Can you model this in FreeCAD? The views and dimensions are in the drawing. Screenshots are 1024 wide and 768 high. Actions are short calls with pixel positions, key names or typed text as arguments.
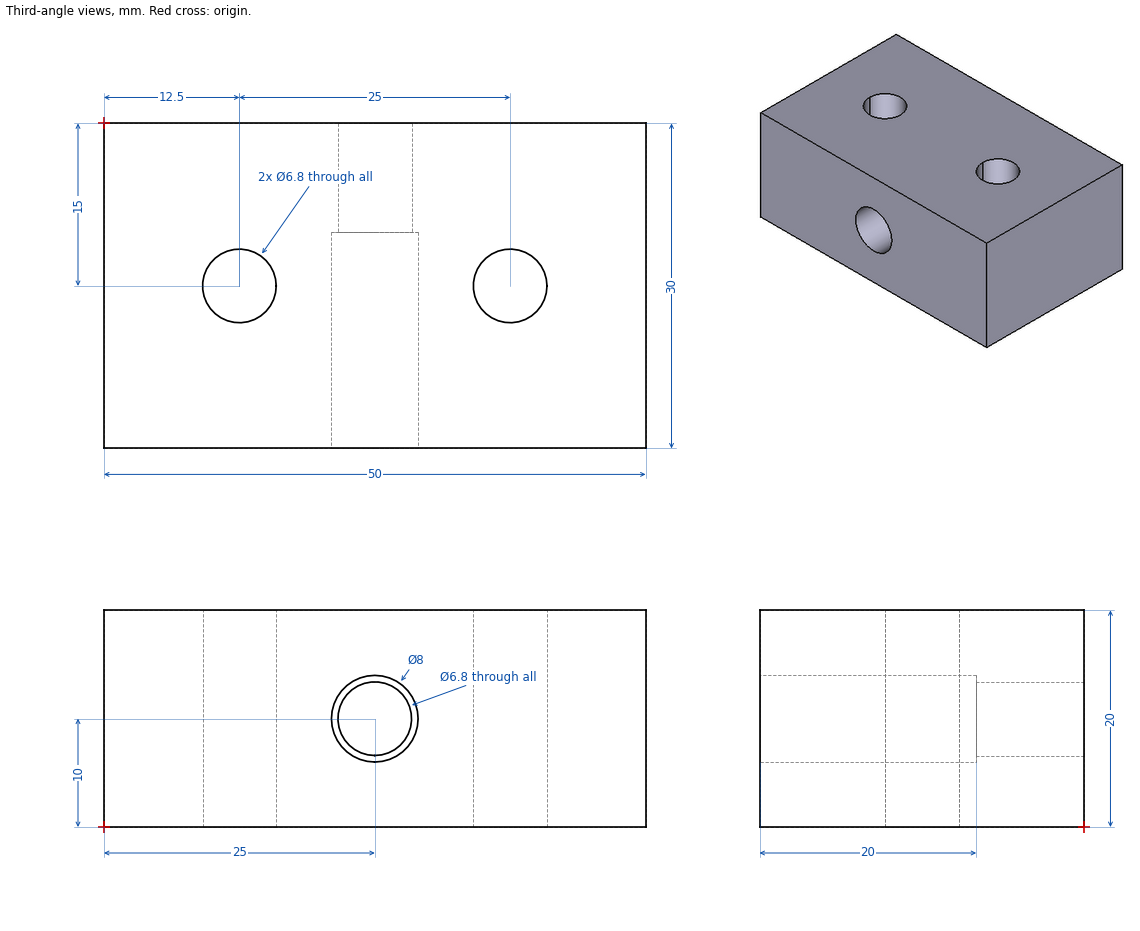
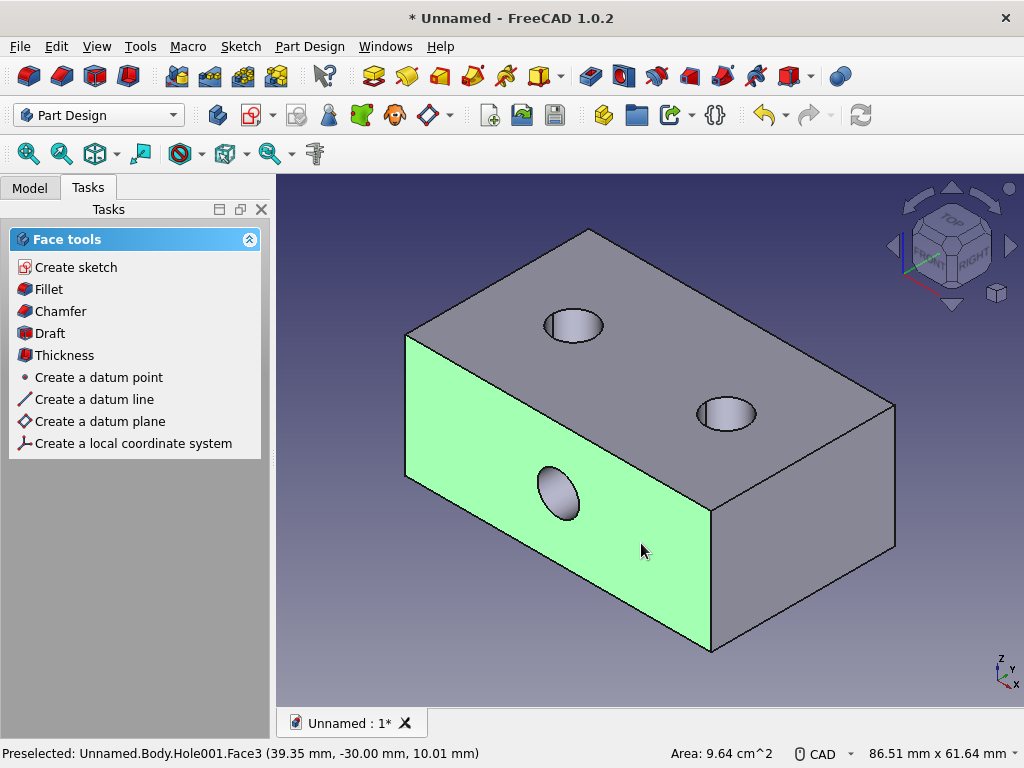
click(250, 116)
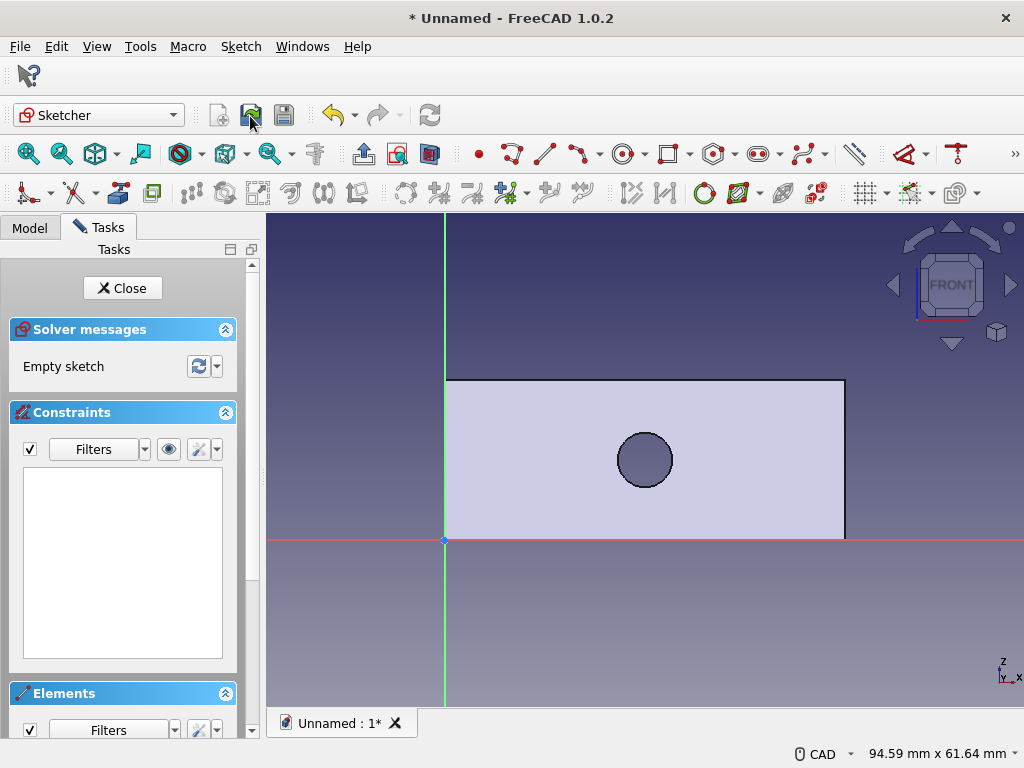
scroll(662, 460, up, 8)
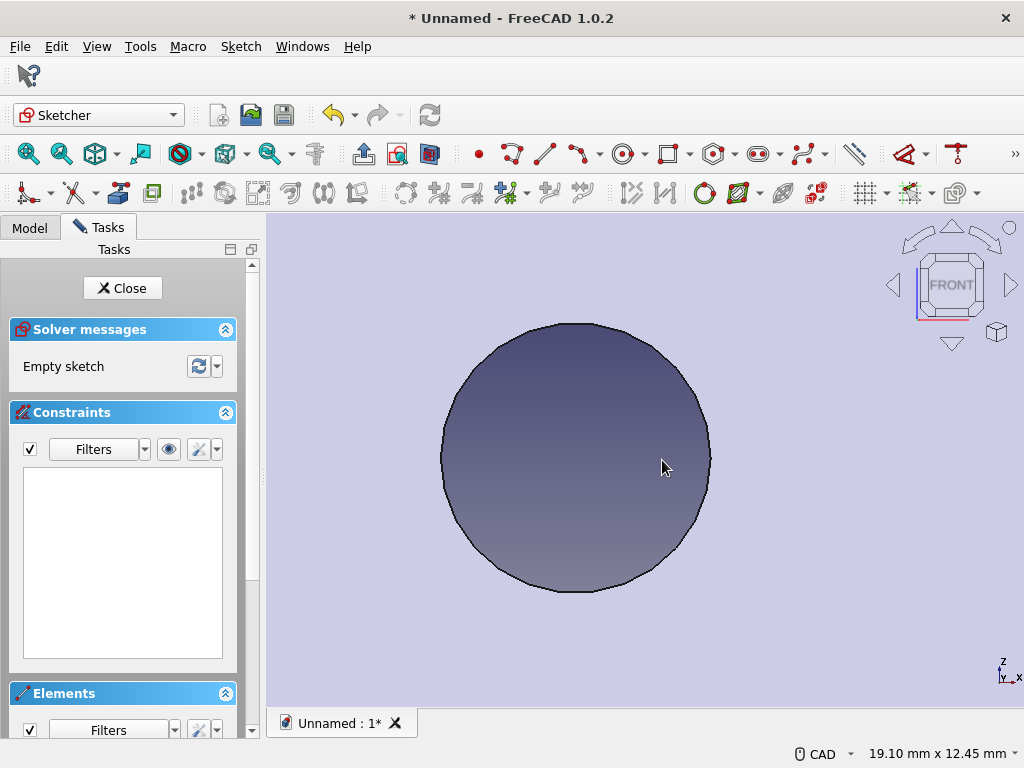
click(622, 154)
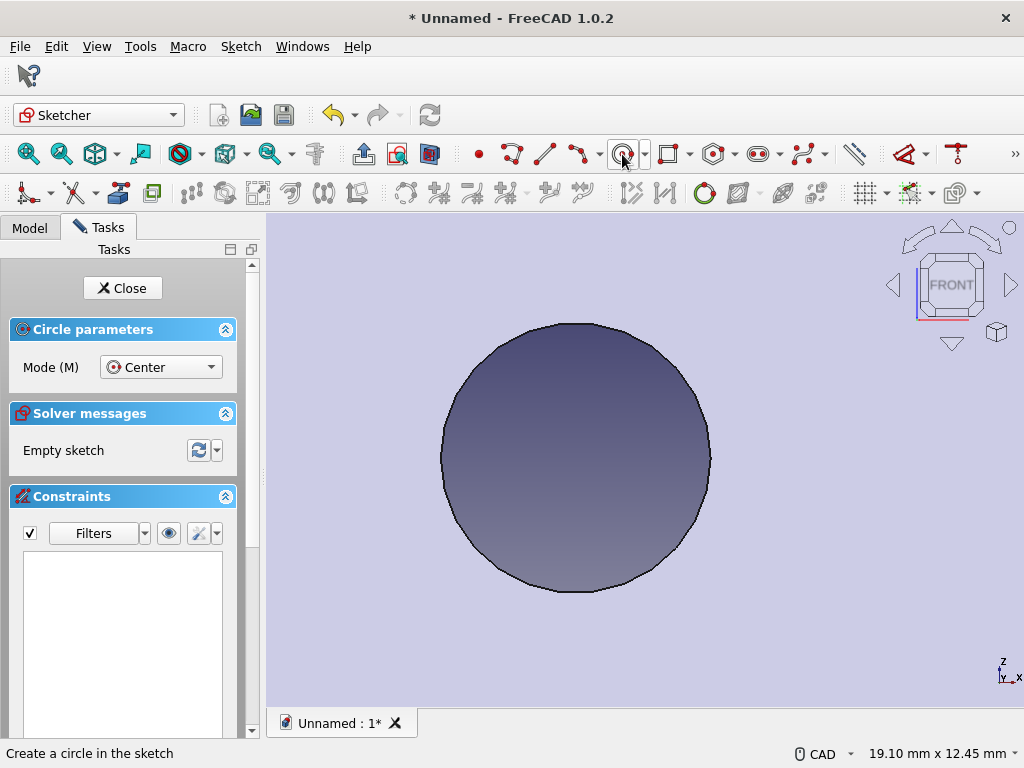
click(576, 458)
move(688, 346)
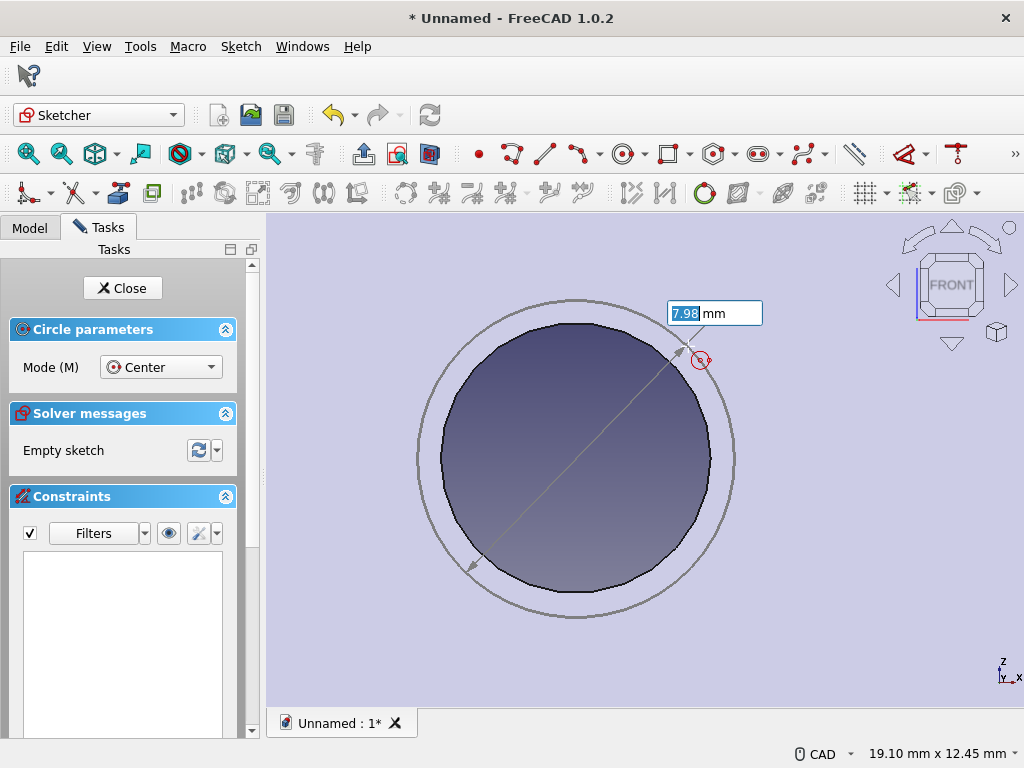
text(8)
key(Return)
key(Escape)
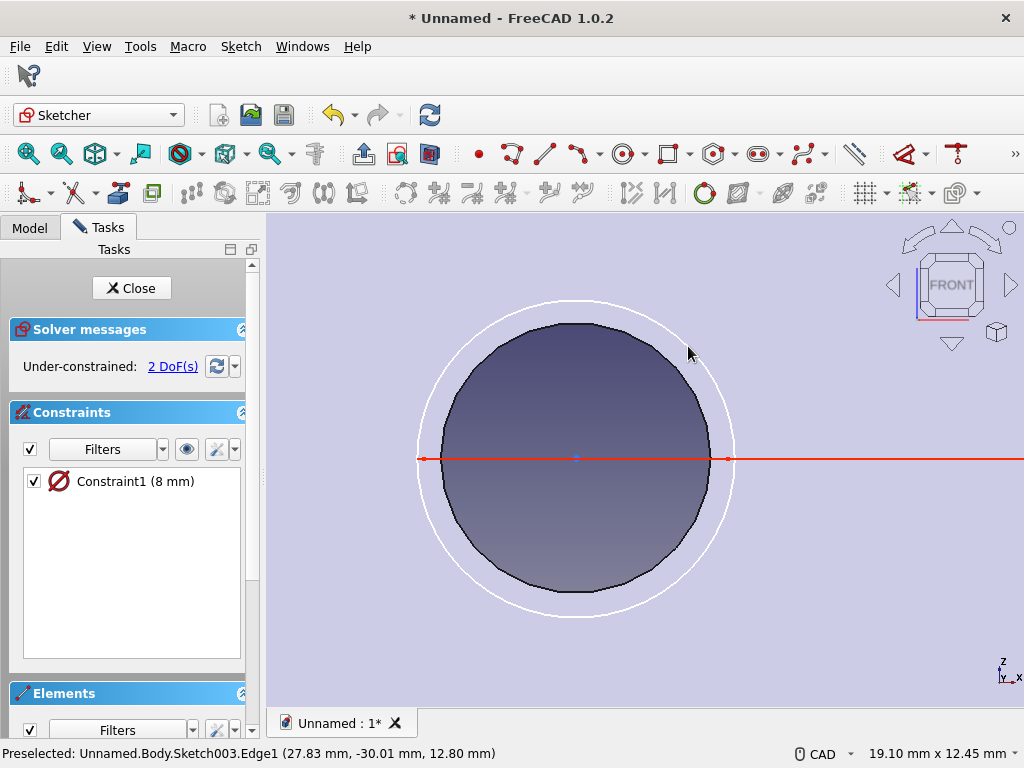
click(904, 154)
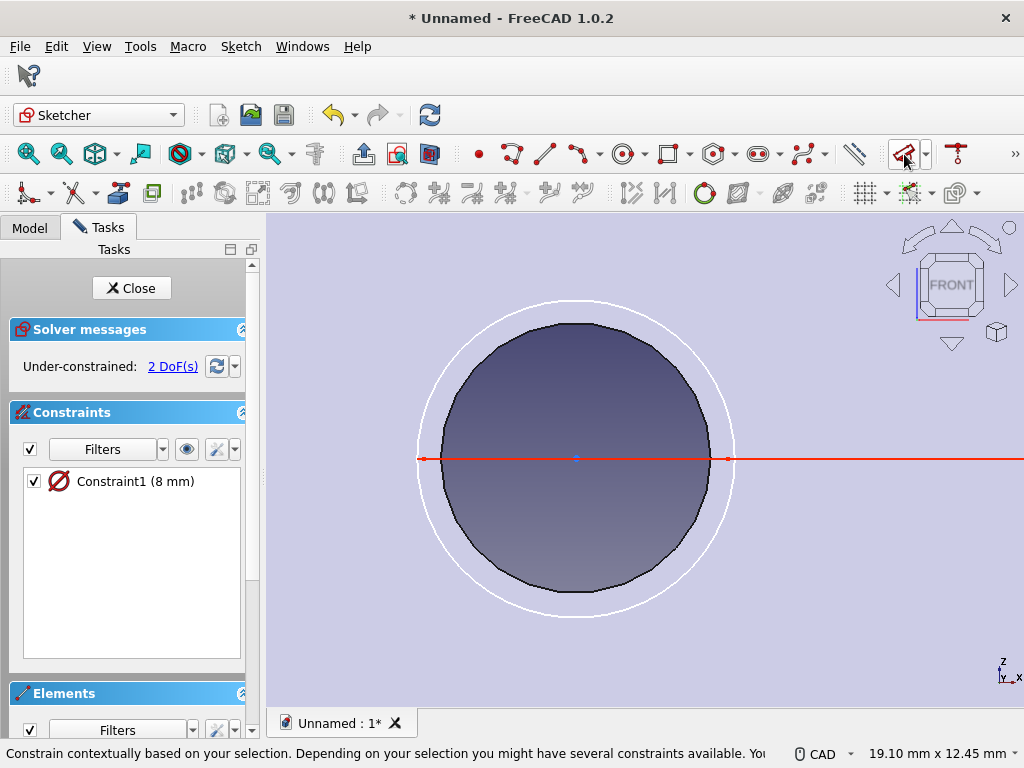
click(576, 459)
click(435, 425)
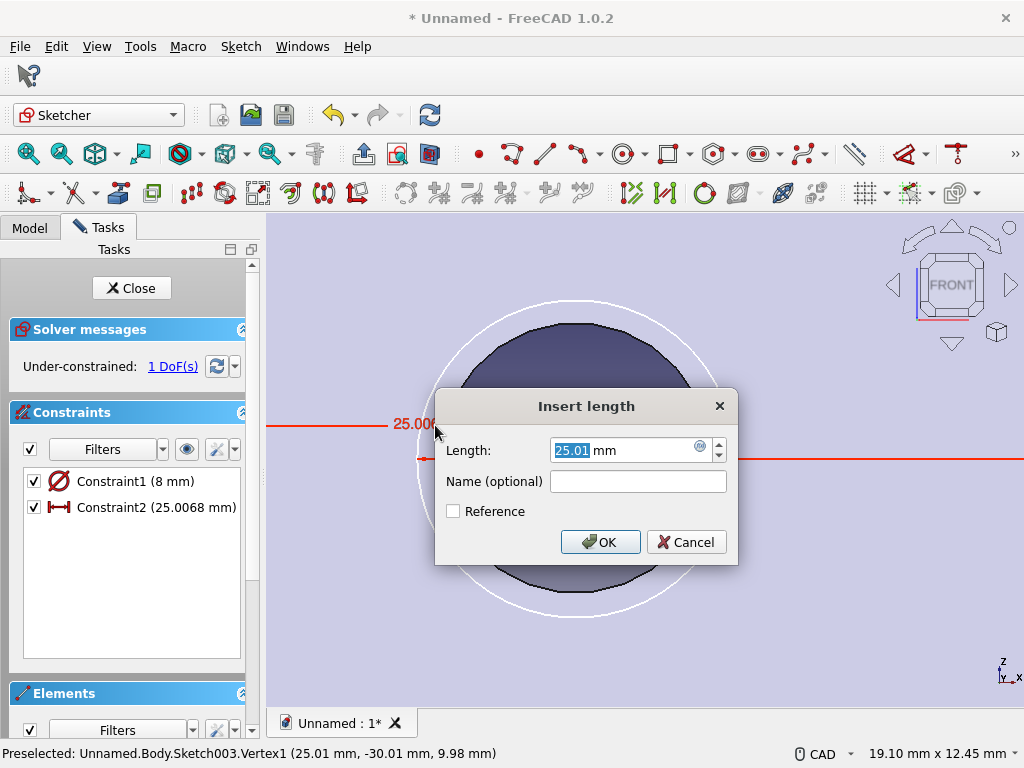
text(25)
key(Return)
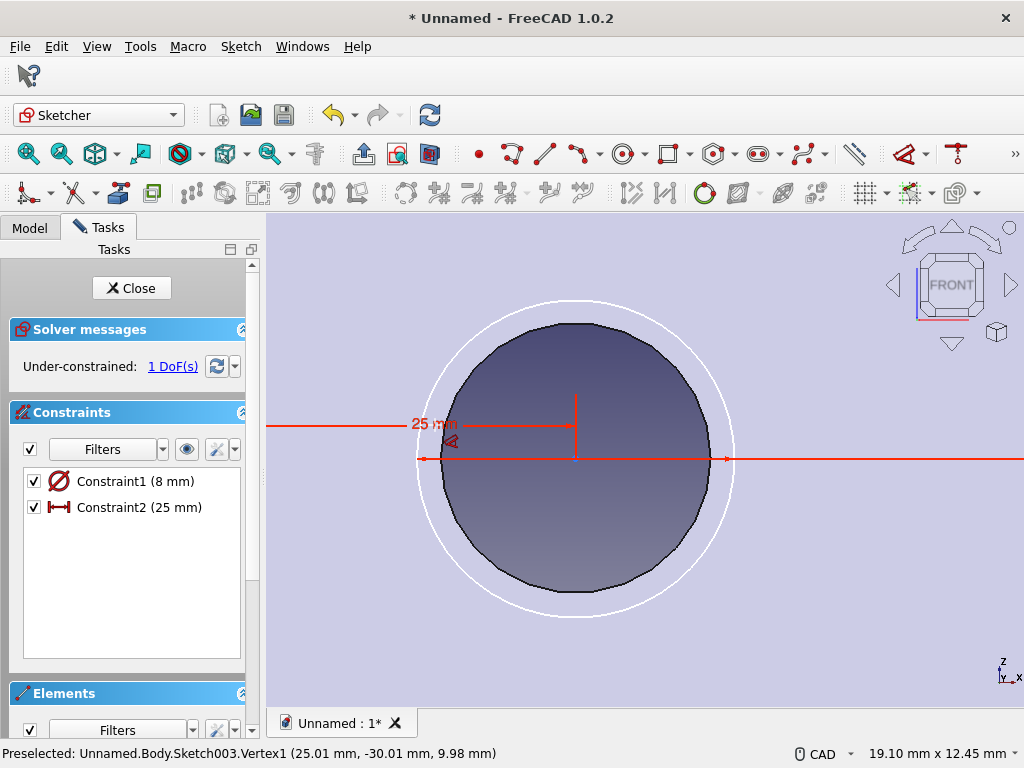
click(576, 459)
click(610, 569)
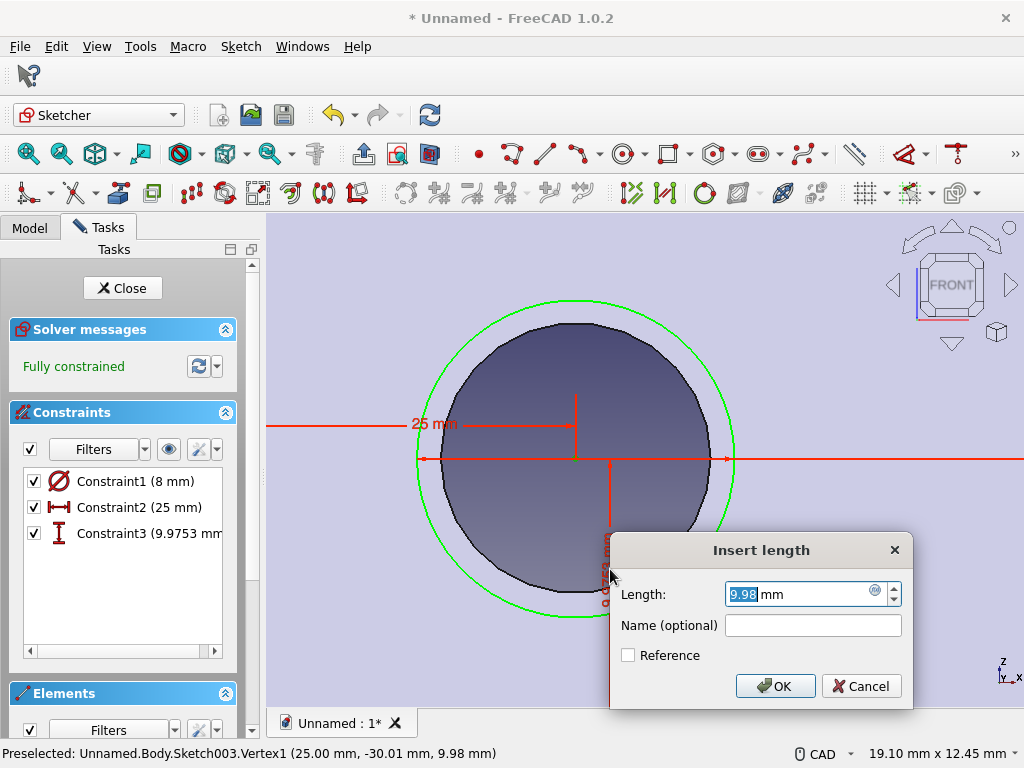
text(10)
key(Return)
key(Escape)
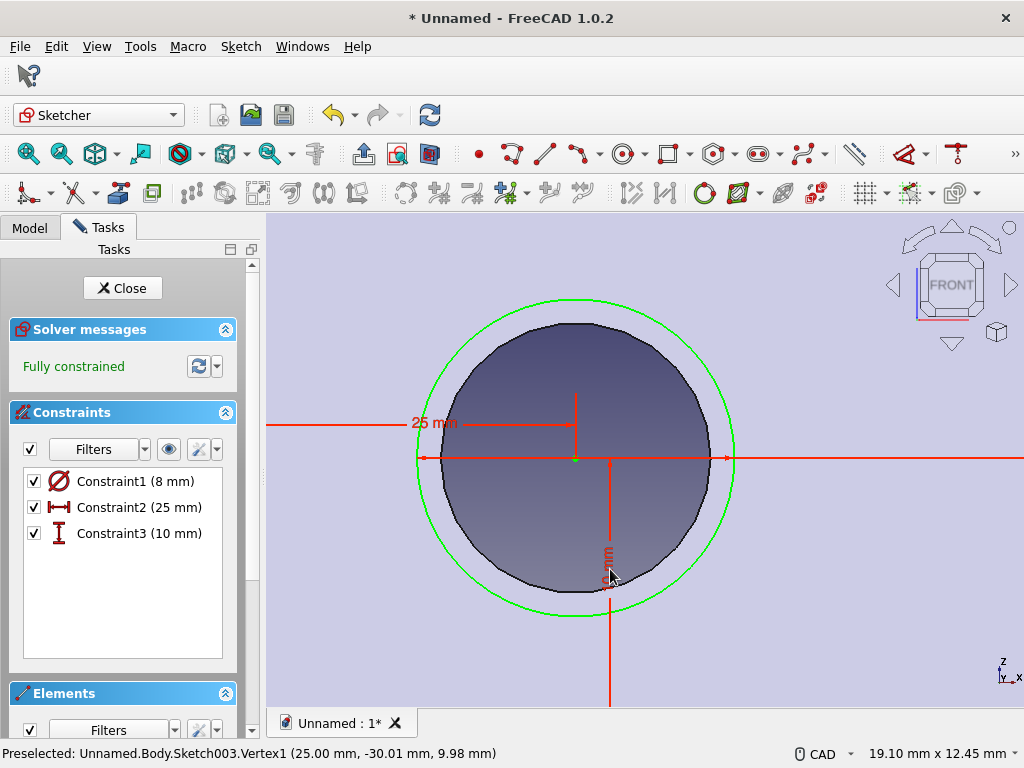
click(123, 288)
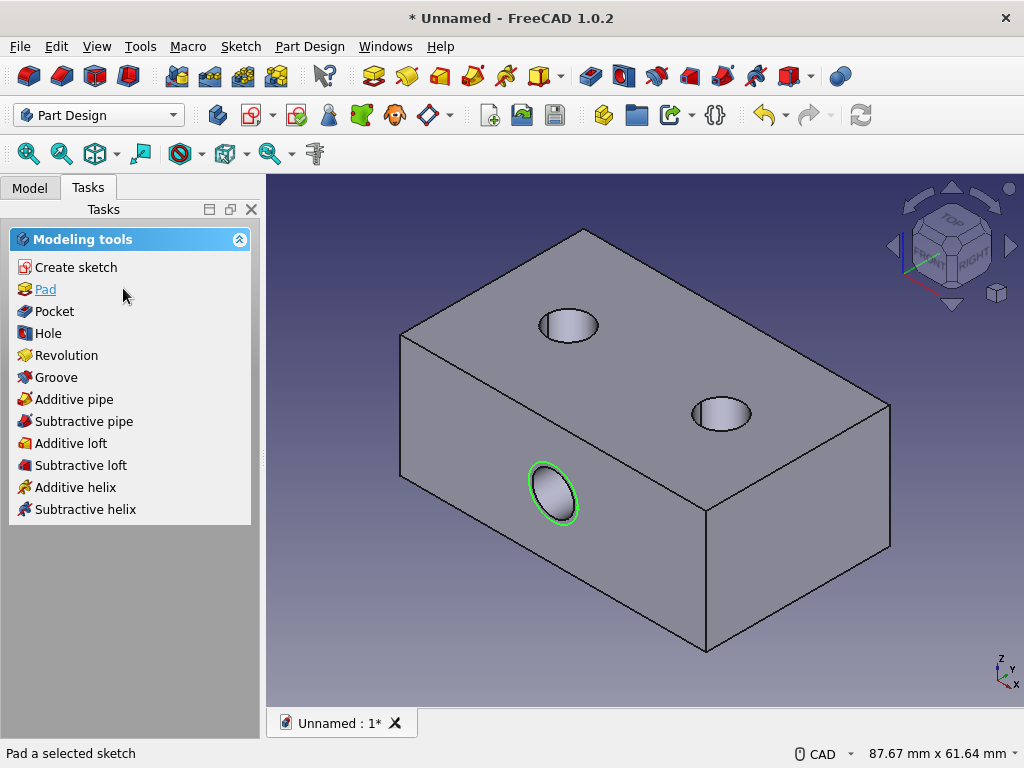
click(591, 76)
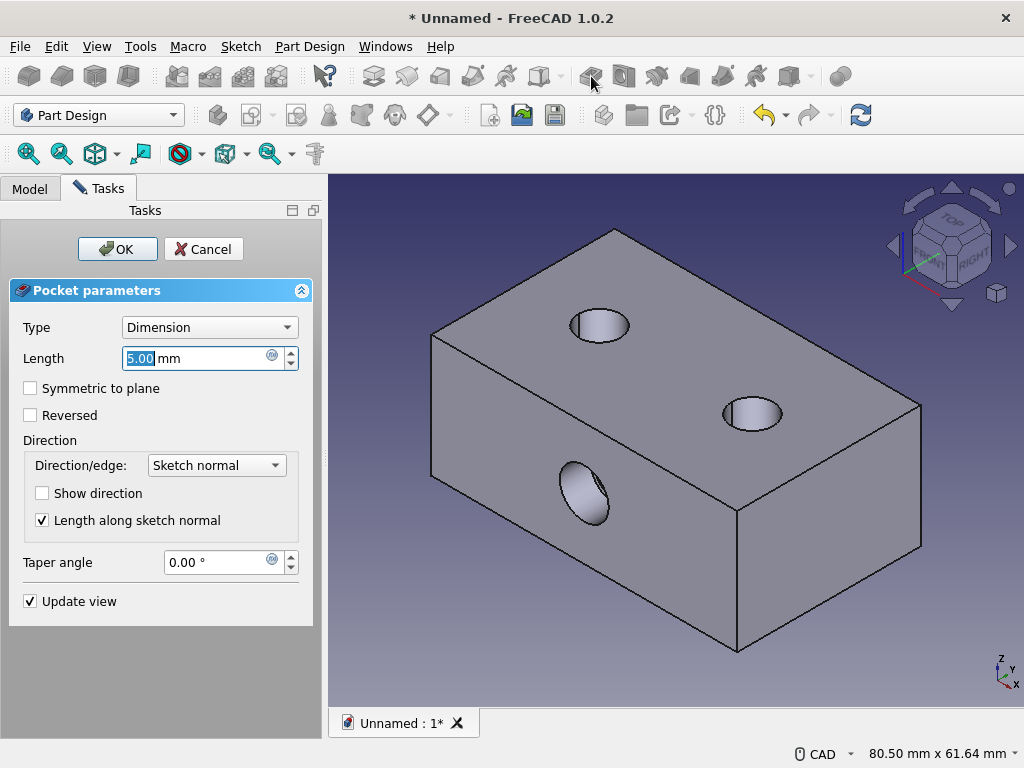
text(20)
key(Tab)